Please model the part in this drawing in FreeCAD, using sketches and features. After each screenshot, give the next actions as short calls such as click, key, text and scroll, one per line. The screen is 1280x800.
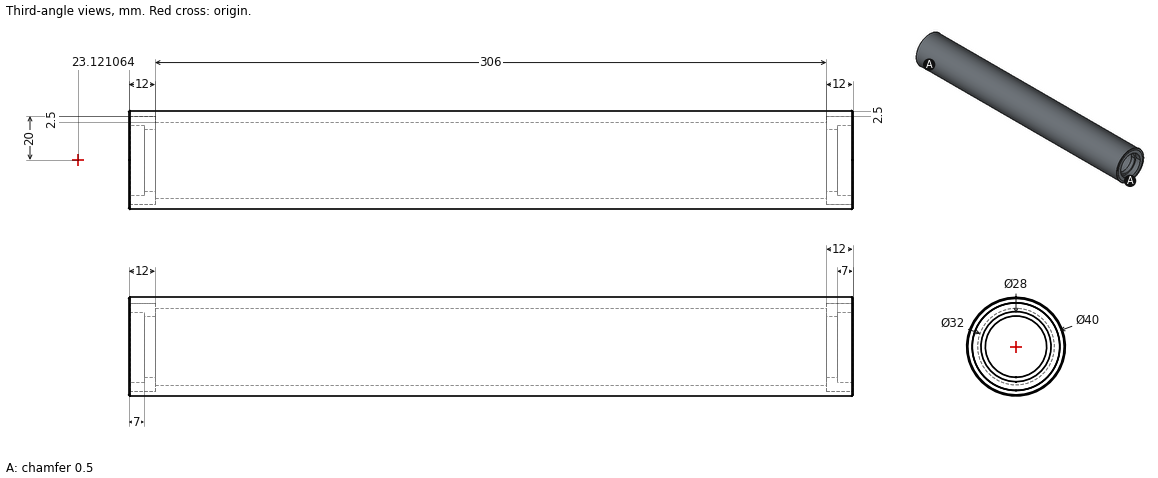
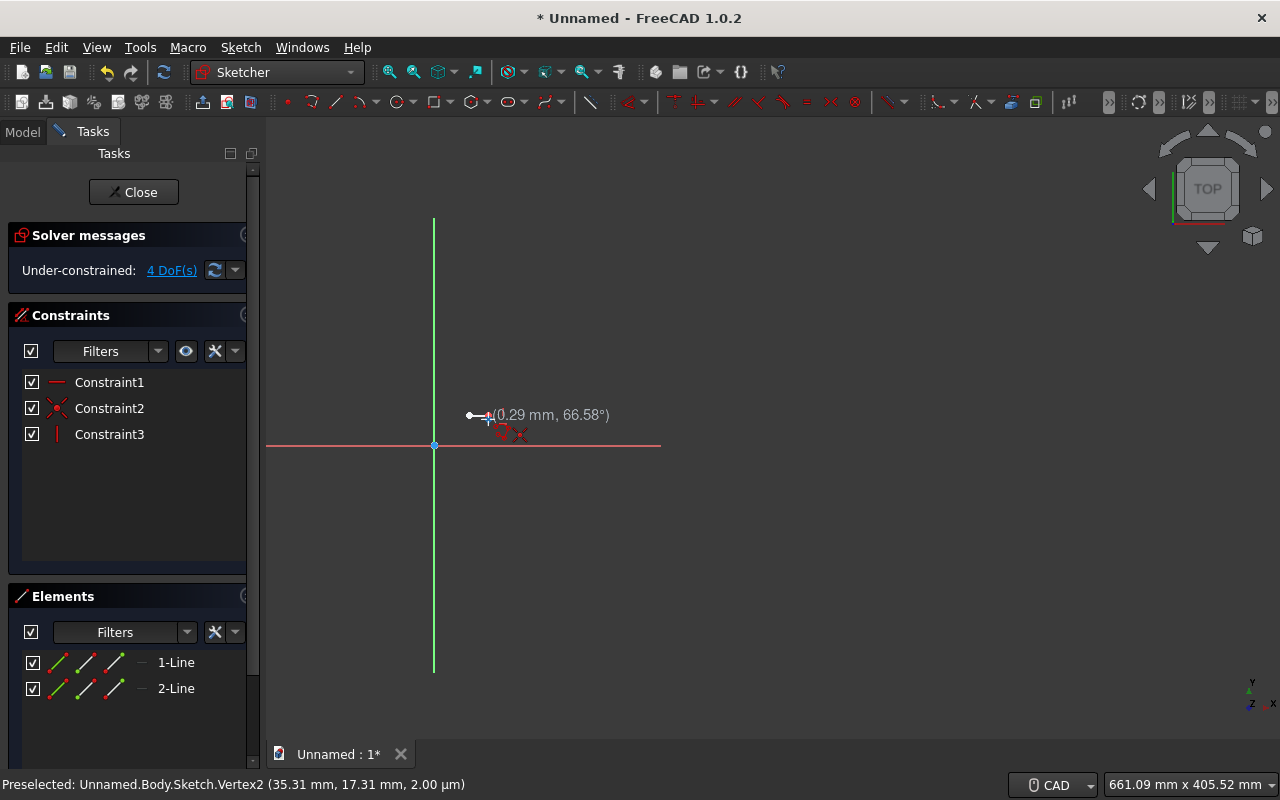
click(957, 419)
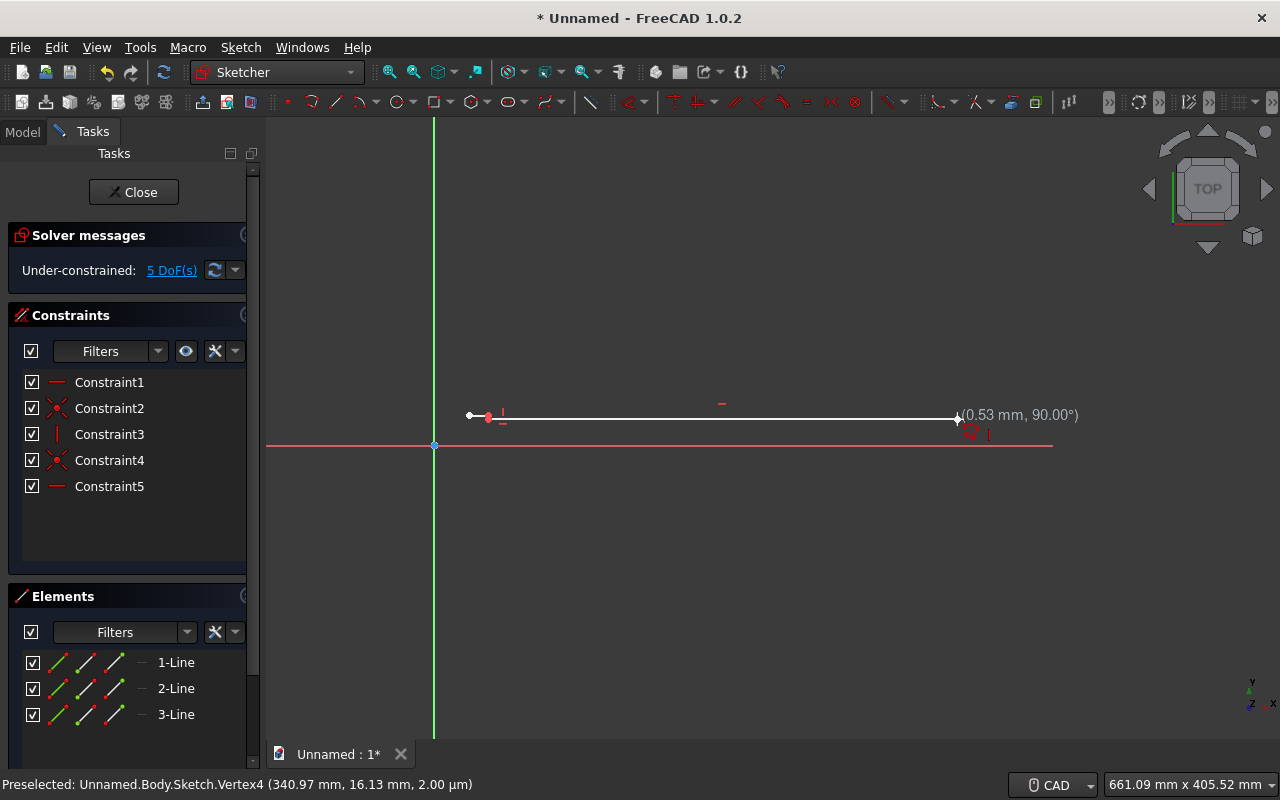
scroll(957, 415, up, 8)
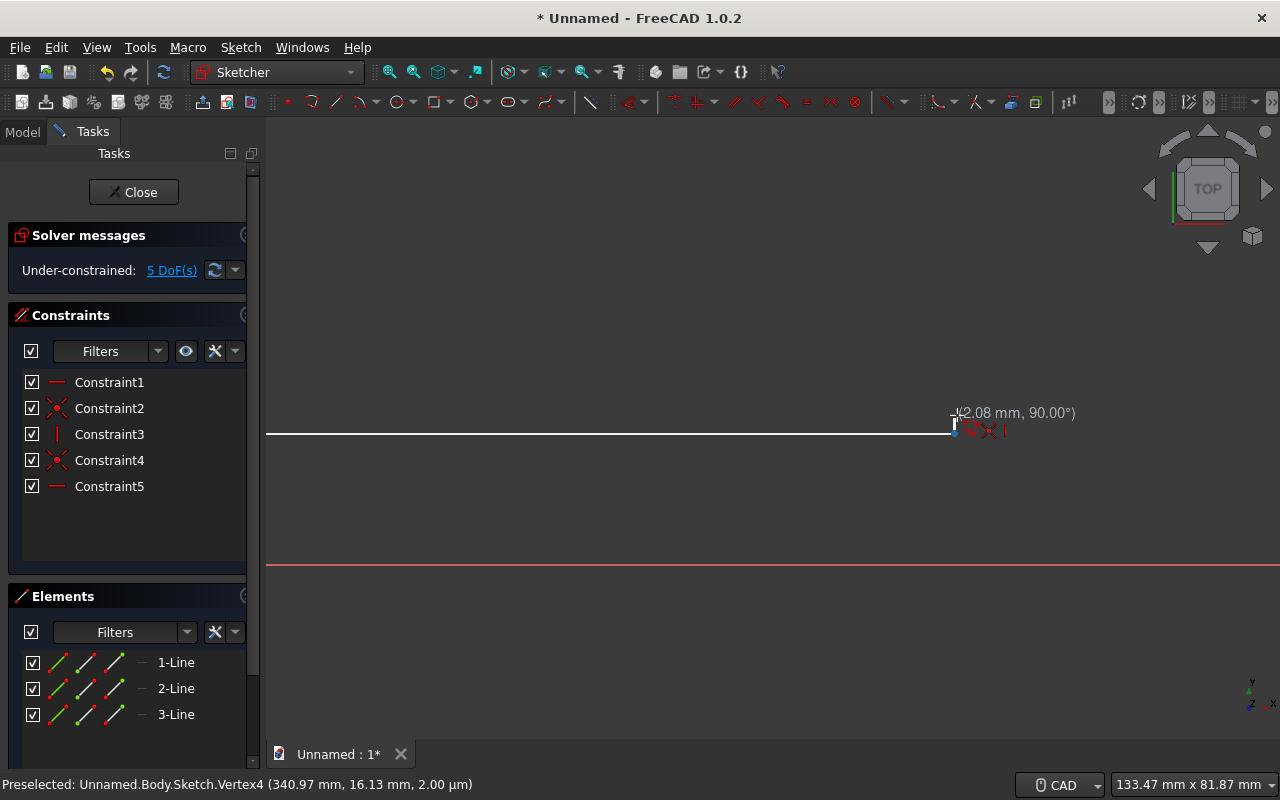
click(954, 413)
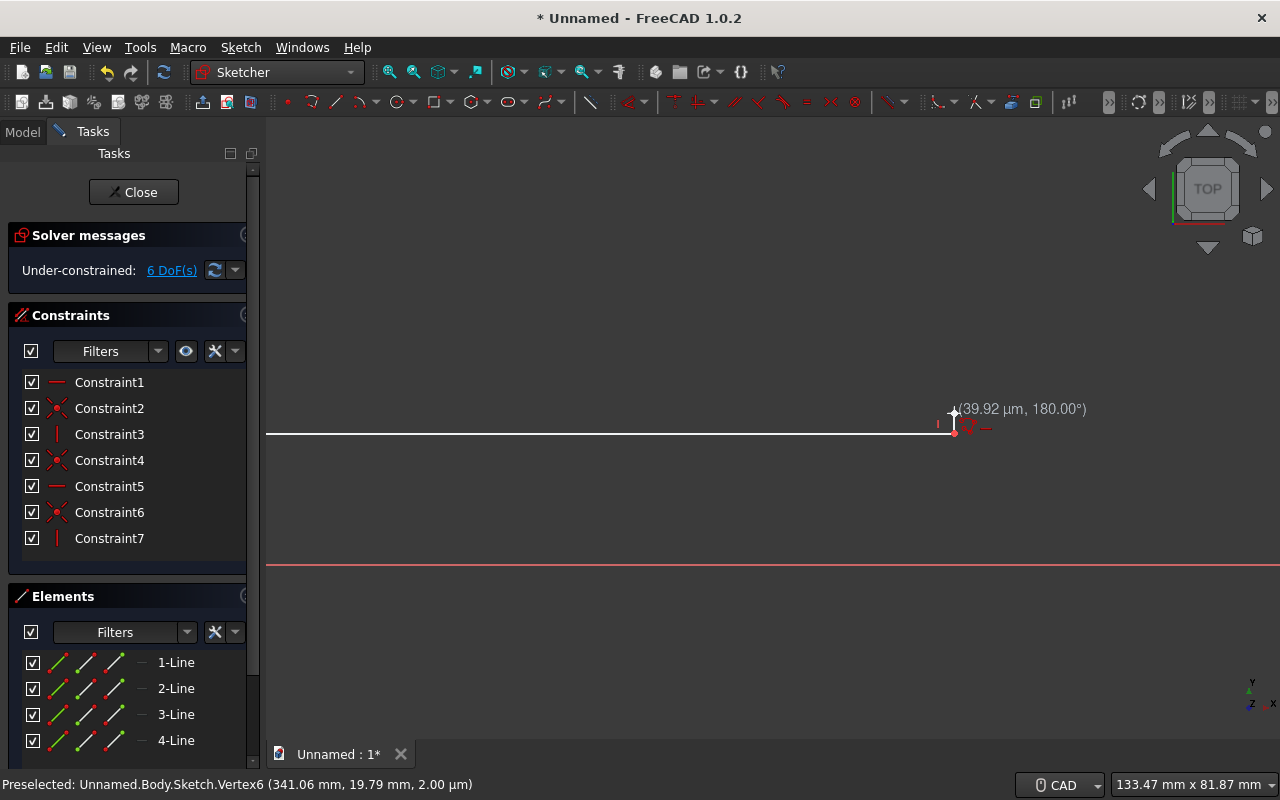
scroll(957, 415, down, 8)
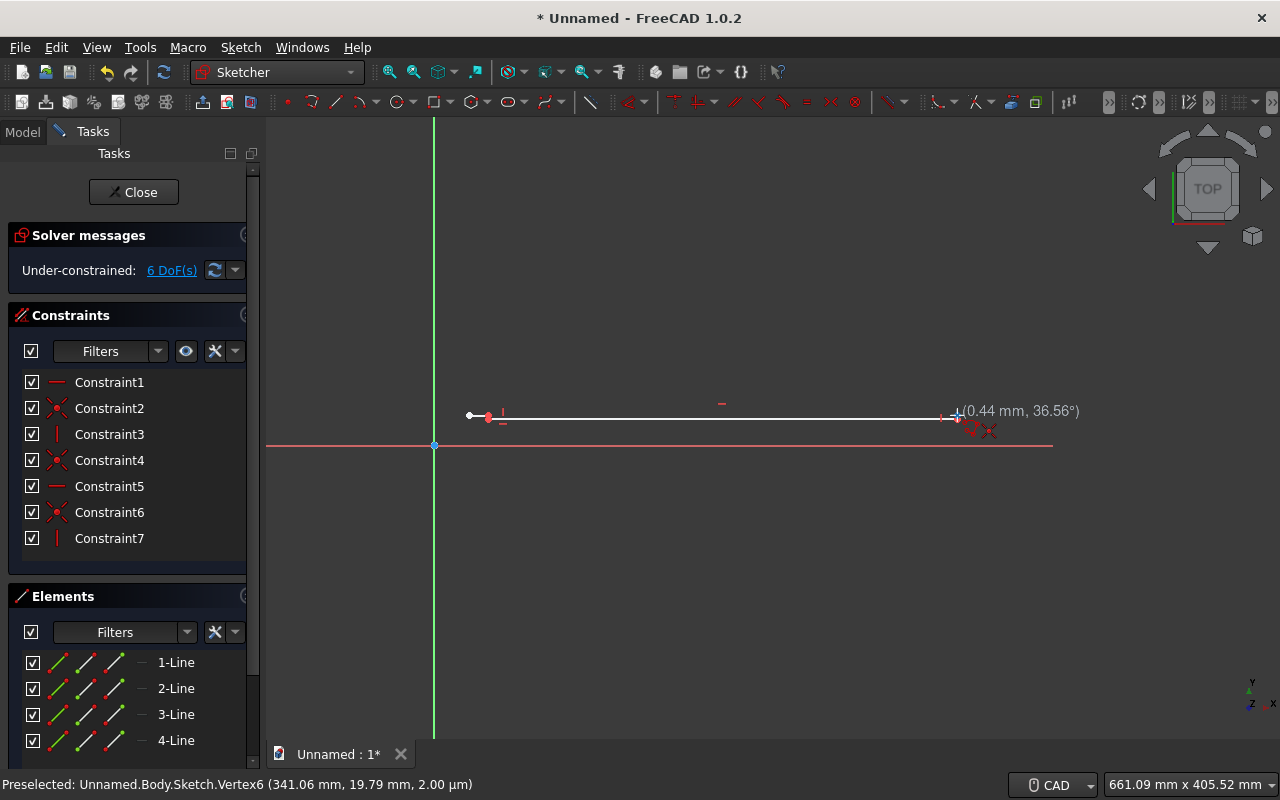
click(976, 415)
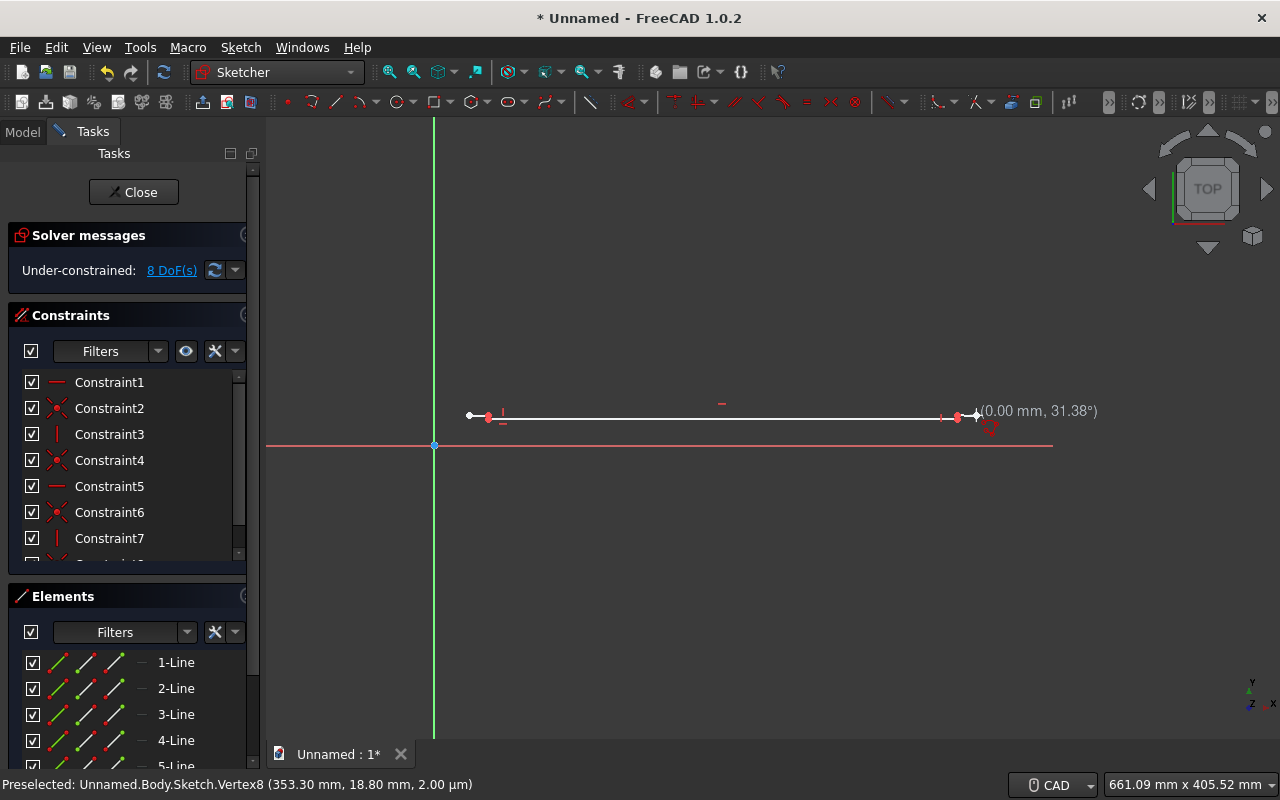
scroll(976, 411, up, 8)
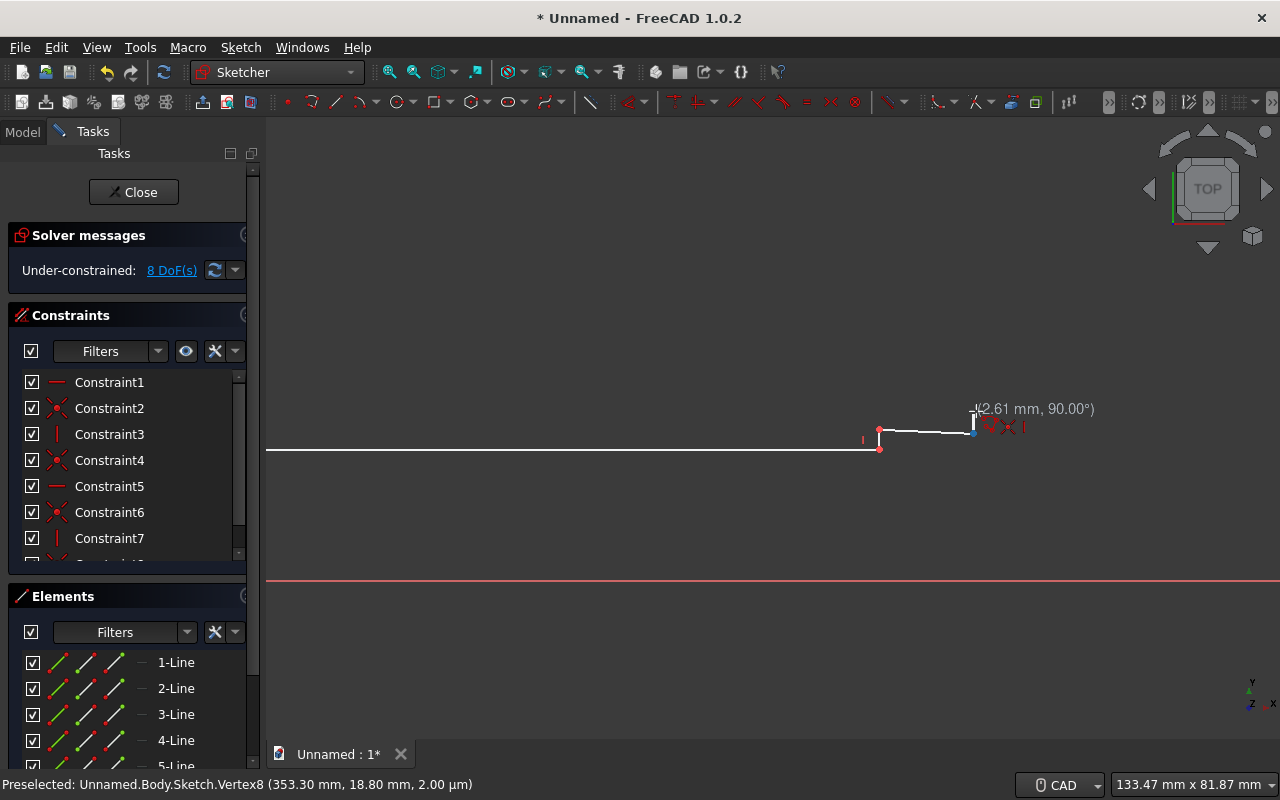
click(973, 410)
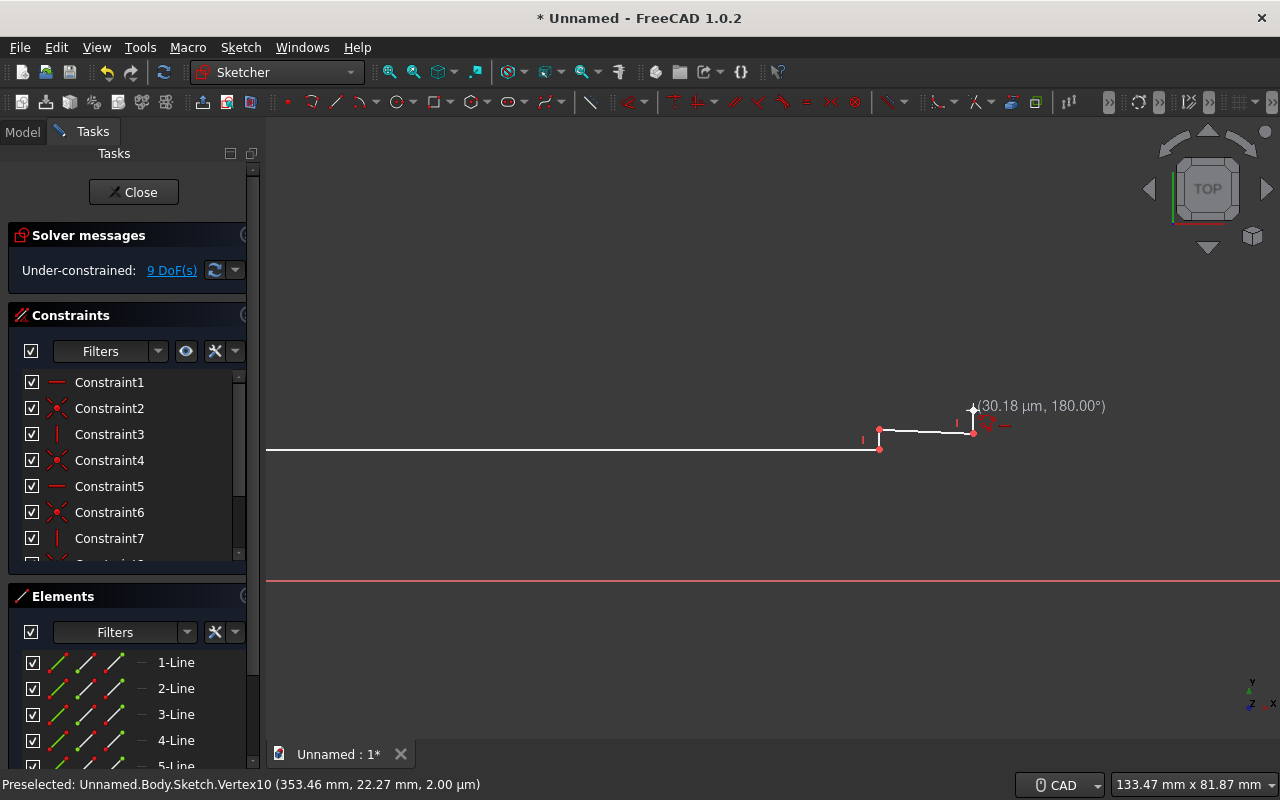
scroll(976, 411, down, 8)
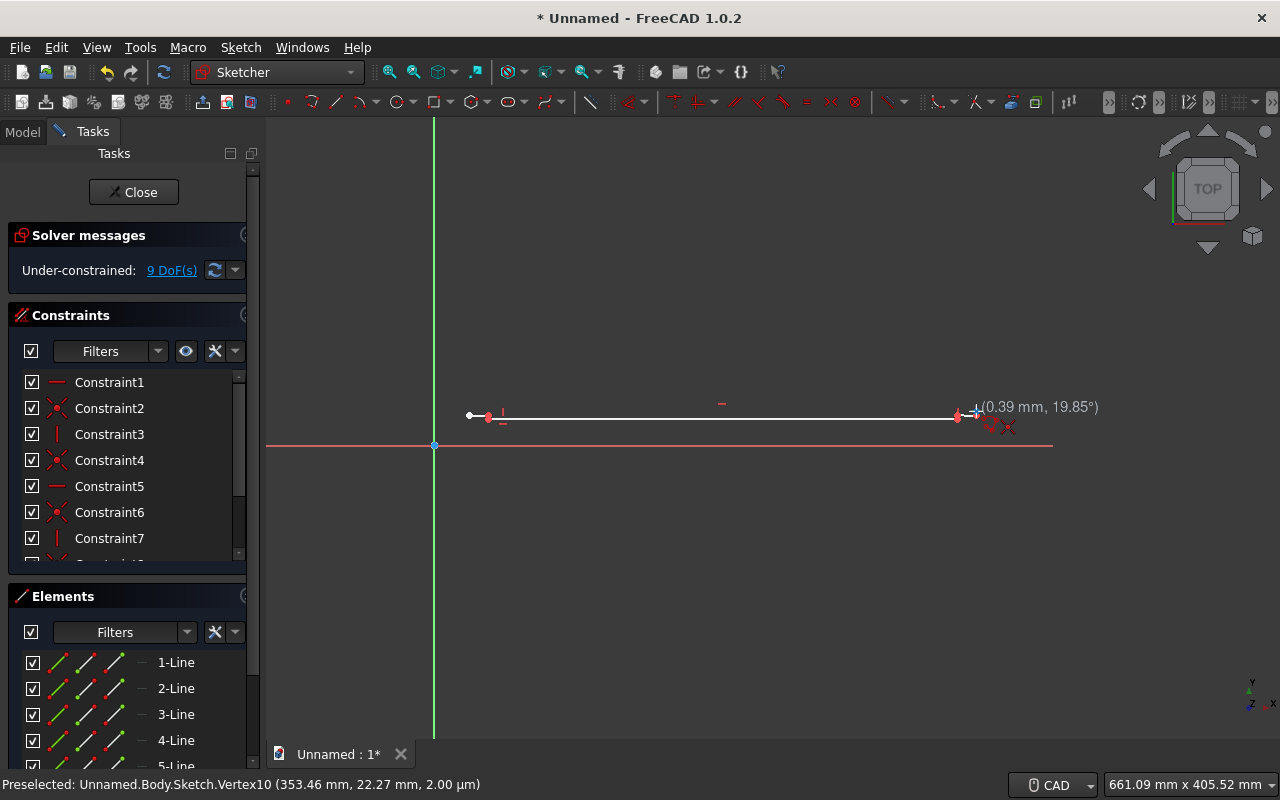
scroll(469, 411, up, 8)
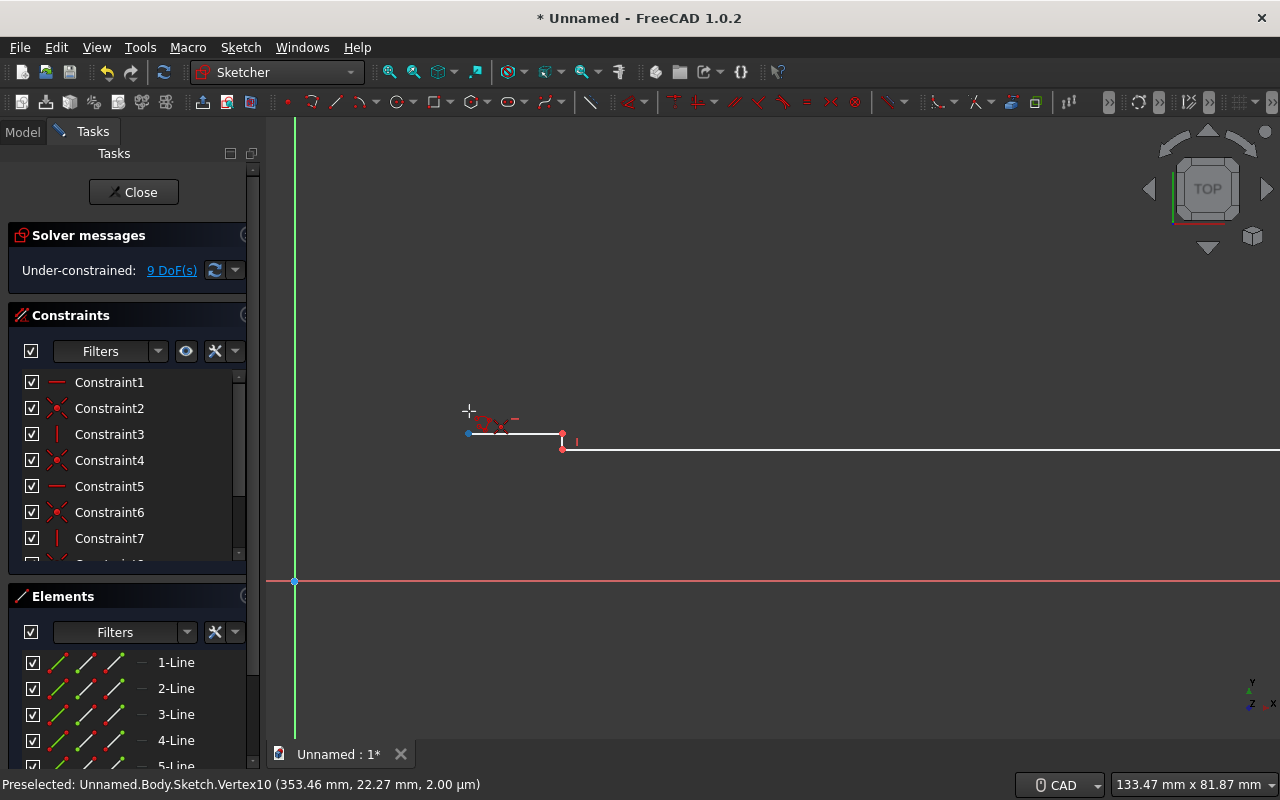
click(471, 410)
click(468, 434)
key(Escape)
key(Escape)